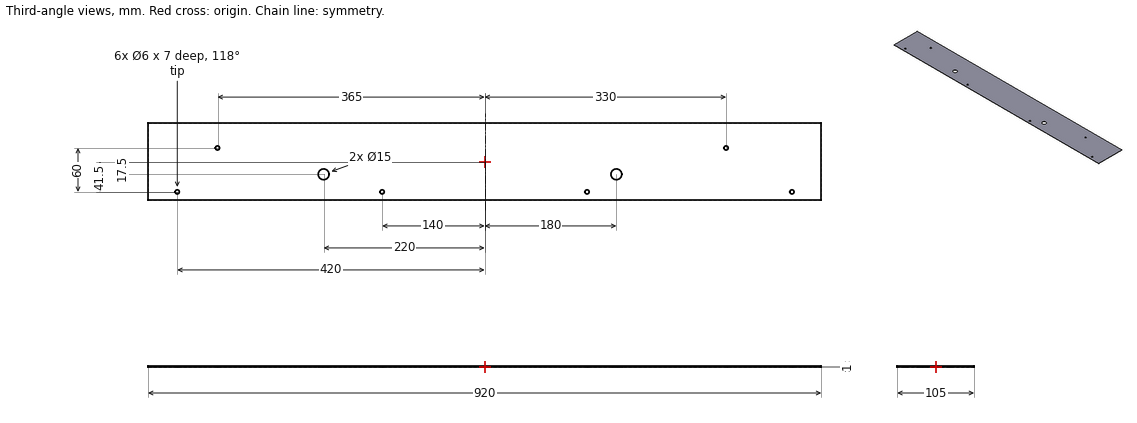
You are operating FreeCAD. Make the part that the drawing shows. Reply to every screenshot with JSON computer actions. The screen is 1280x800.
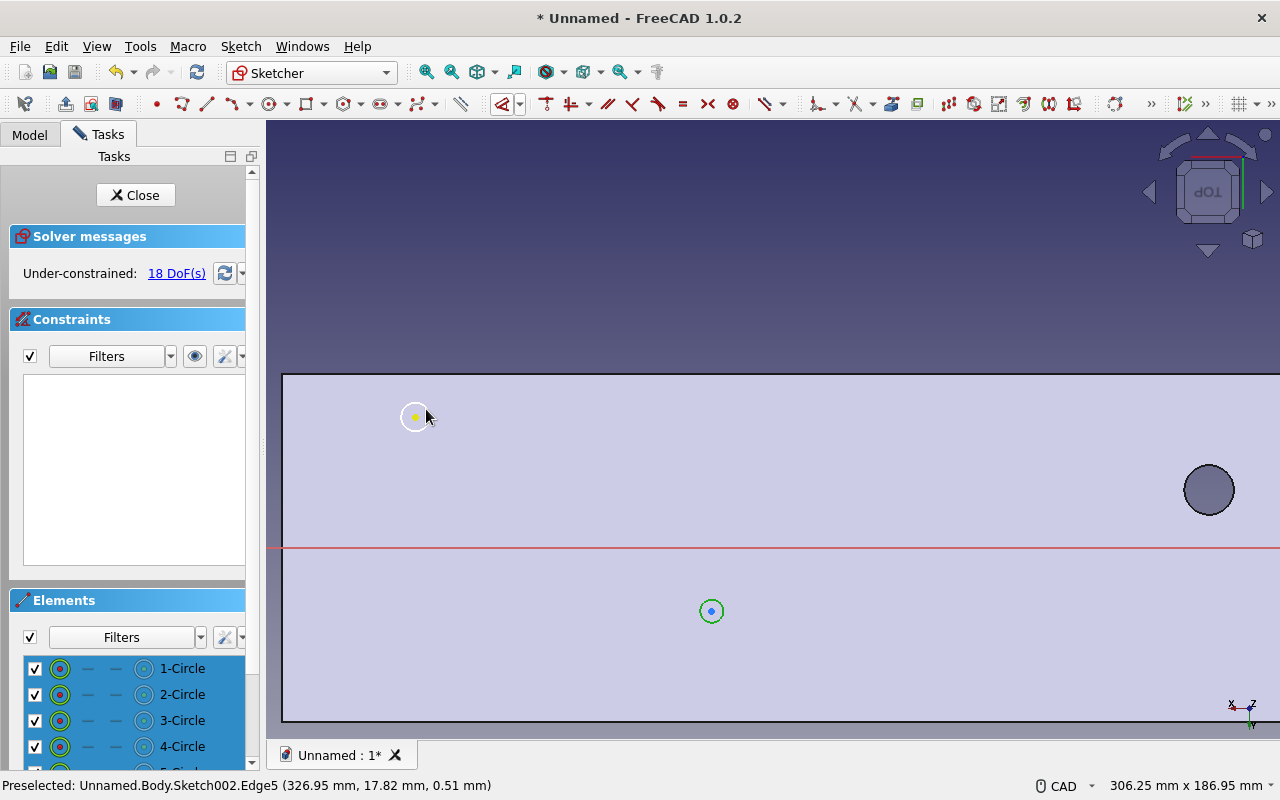
{"action": "left_click", "coordinate": [426, 407]}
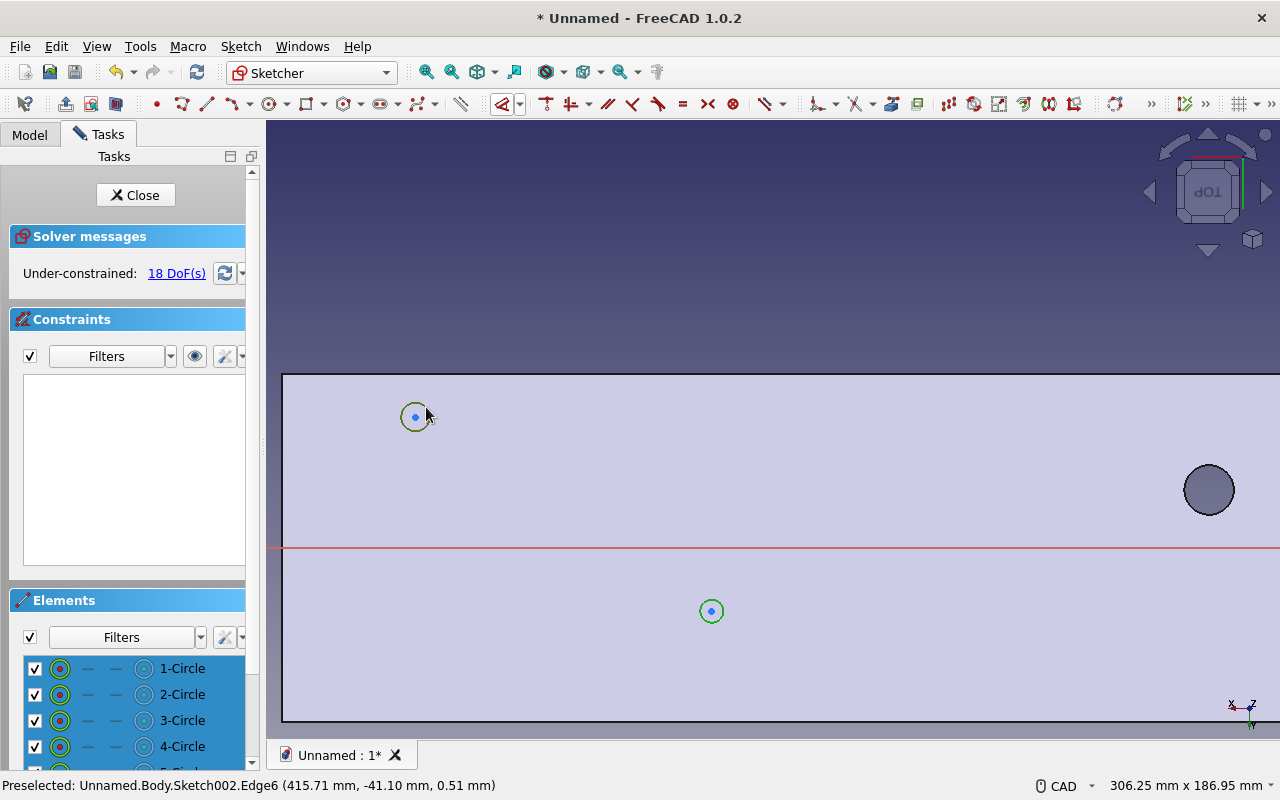
{"action": "left_click", "coordinate": [683, 104]}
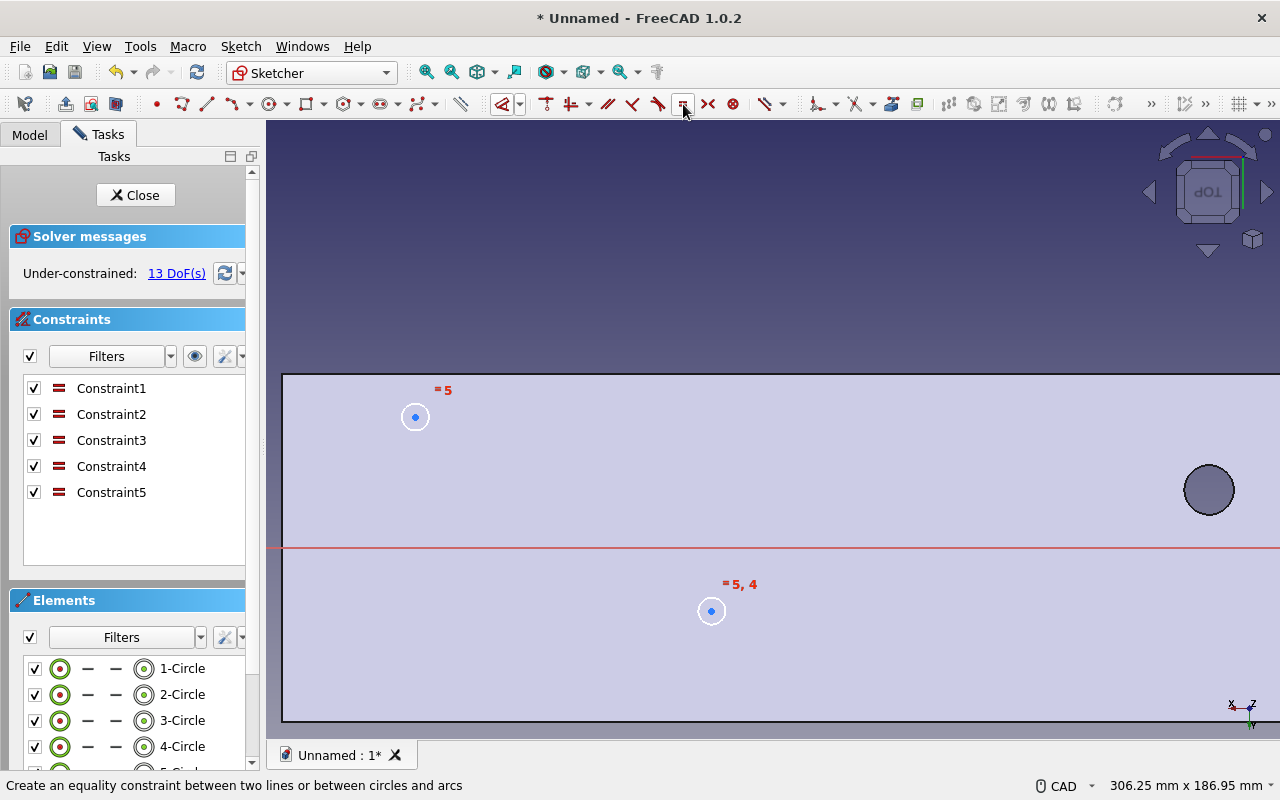
{"action": "scroll", "coordinate": [426, 409], "scroll_direction": "down", "scroll_amount": 8}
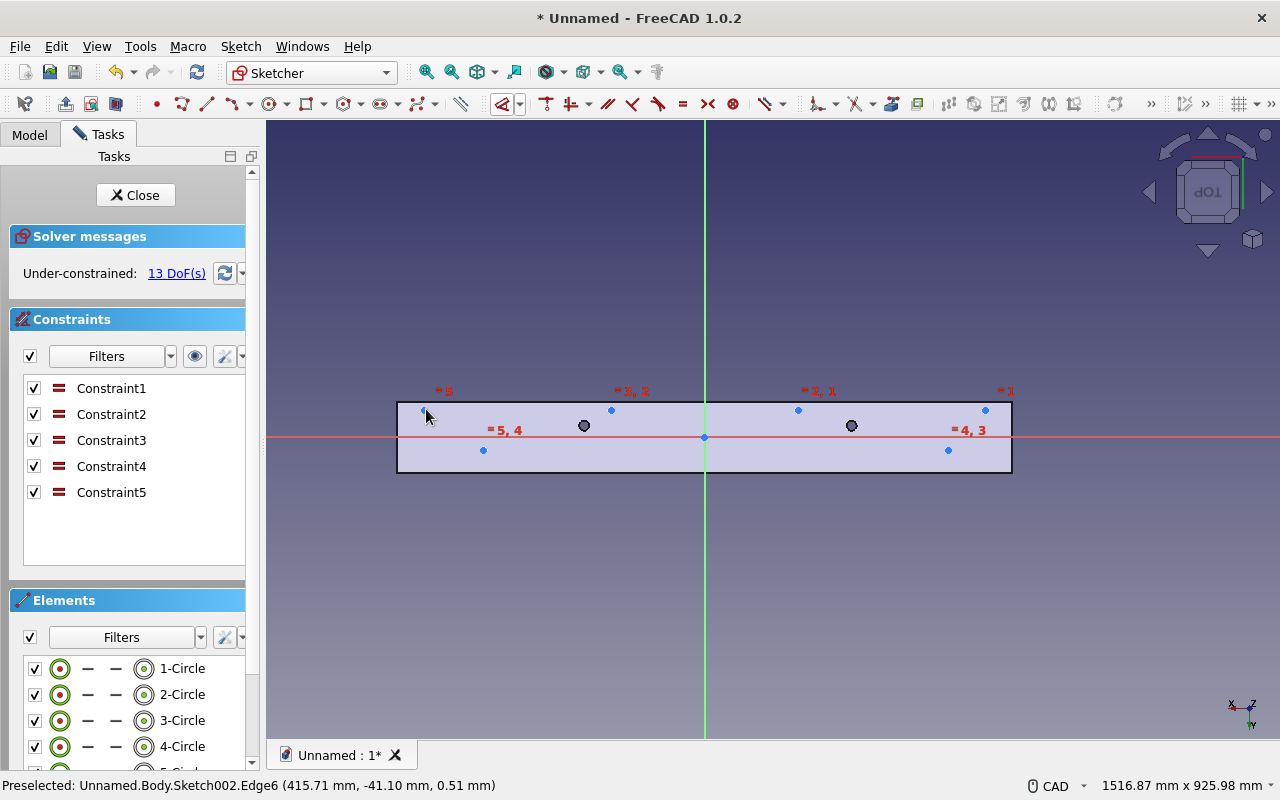
{"action": "left_click", "coordinate": [798, 411]}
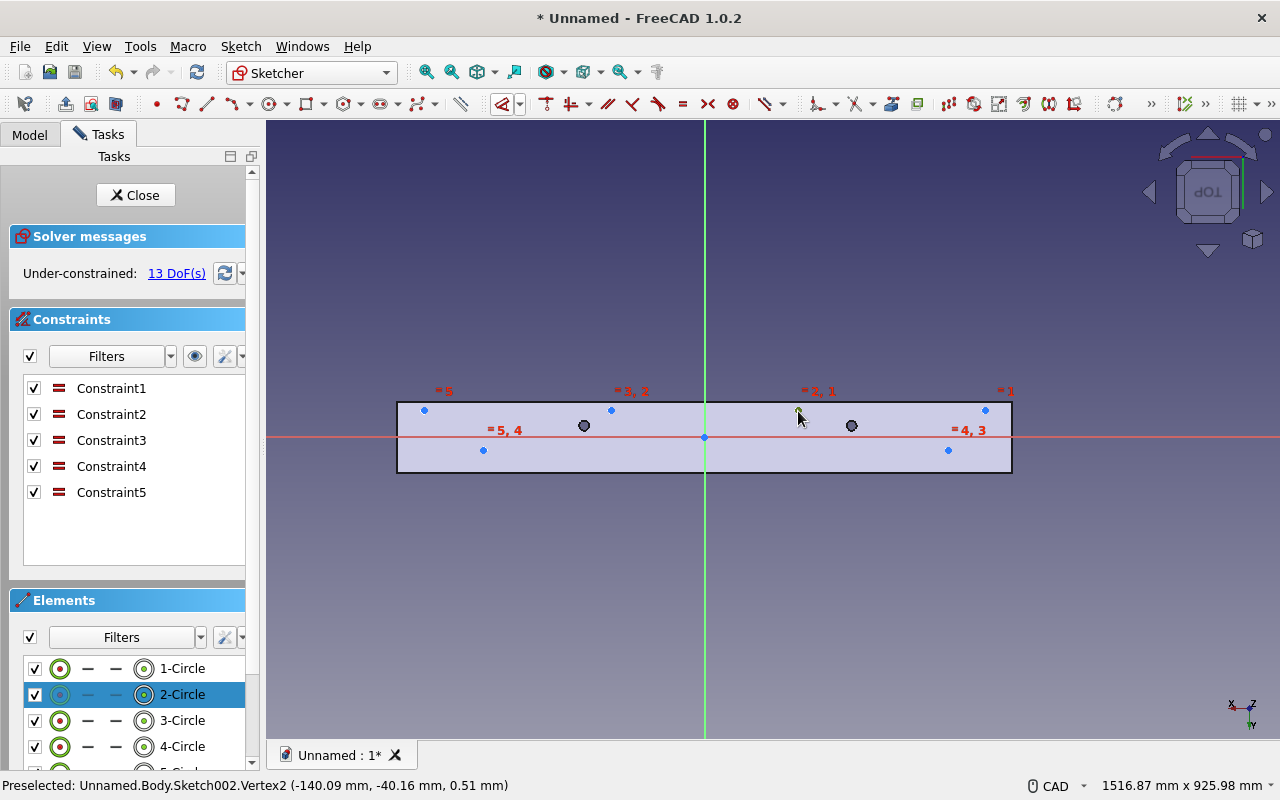
{"action": "left_click", "coordinate": [611, 411]}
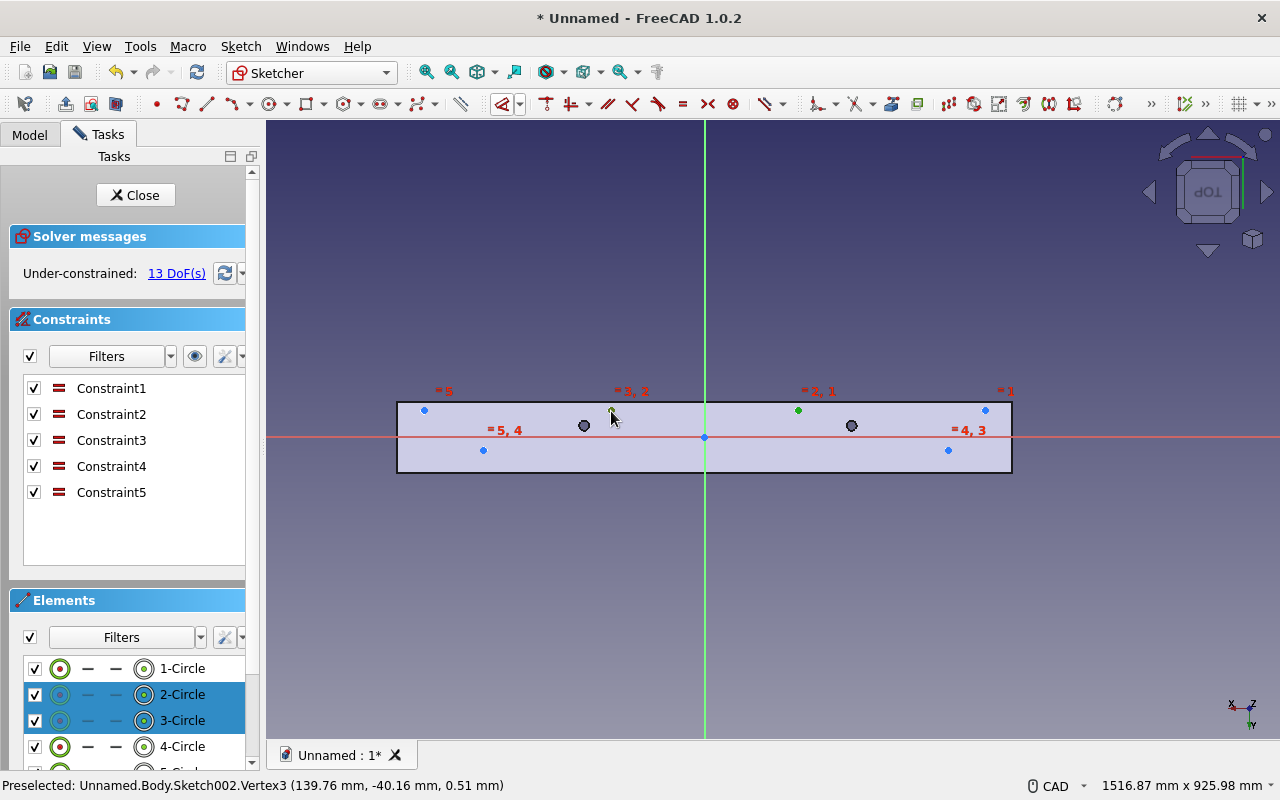
{"action": "left_click", "coordinate": [705, 671]}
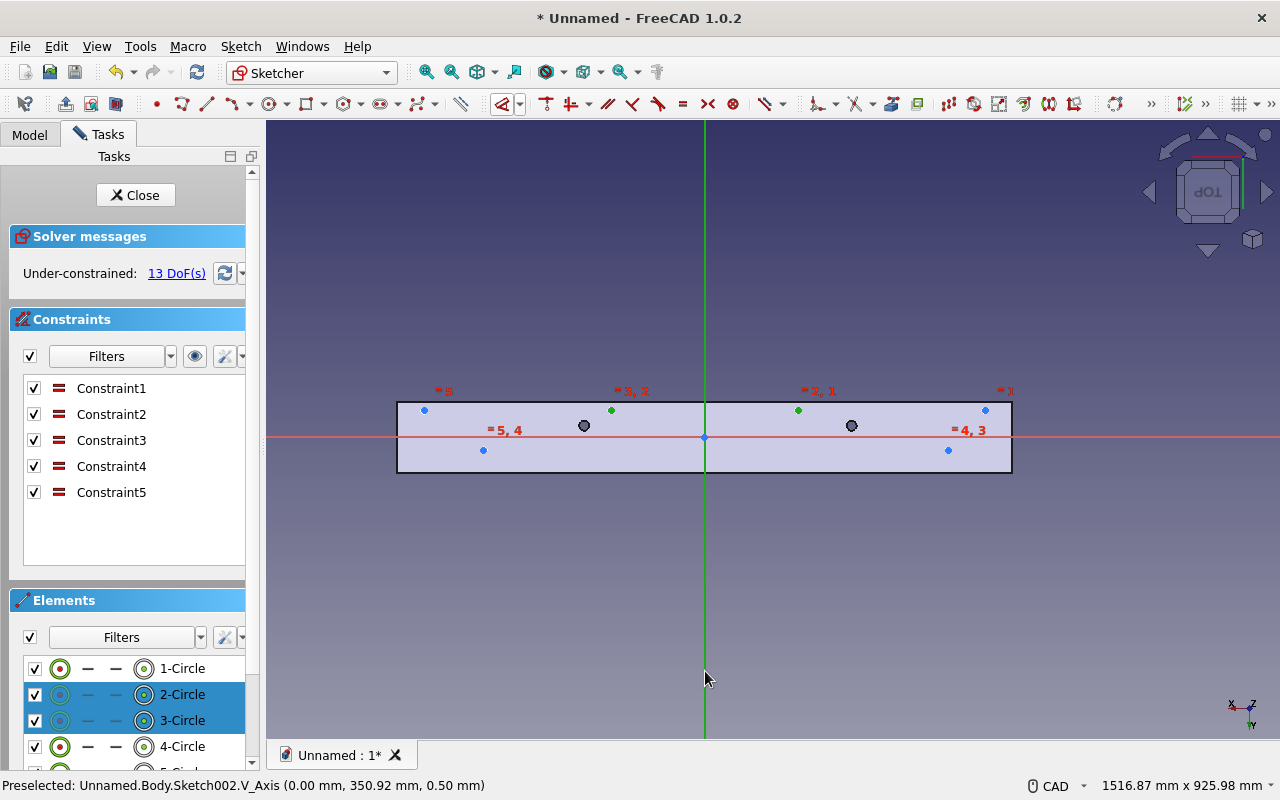
{"action": "left_click", "coordinate": [708, 104]}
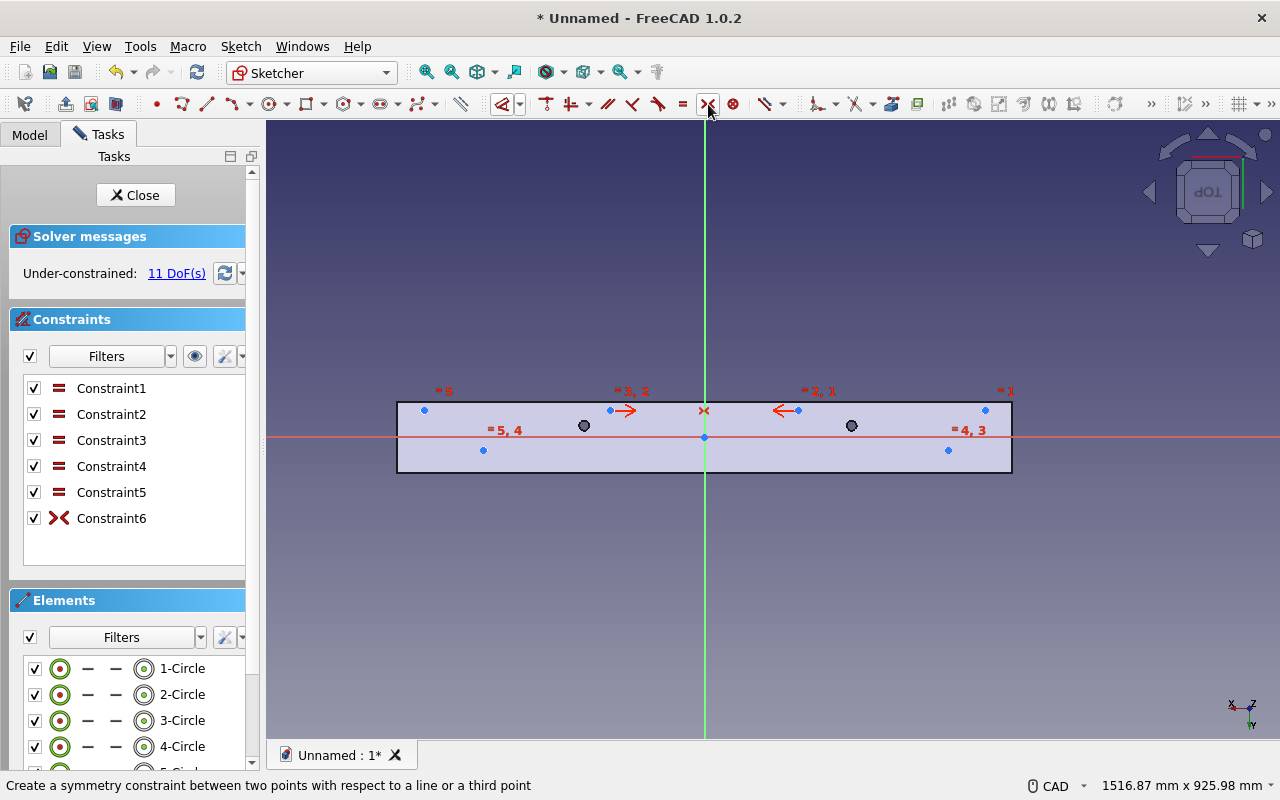
{"action": "left_click", "coordinate": [985, 411]}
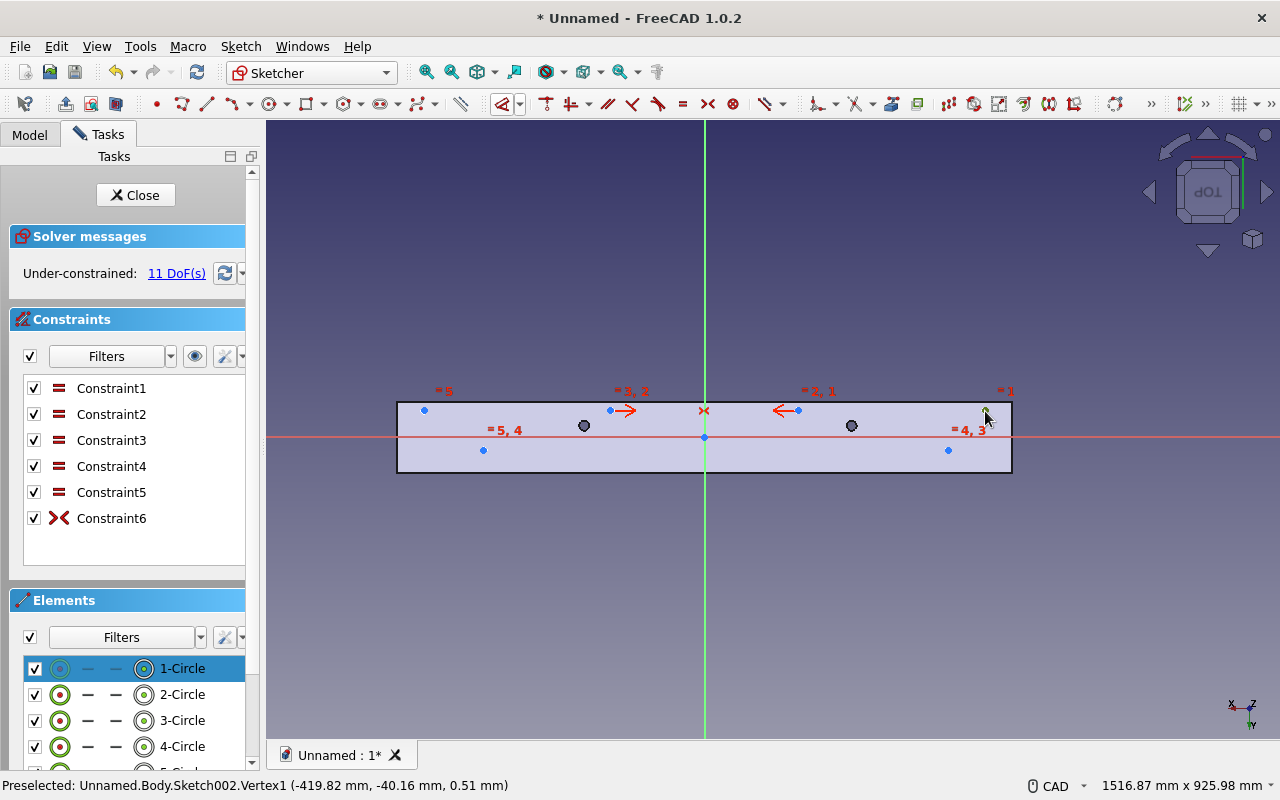
{"action": "left_click", "coordinate": [424, 411]}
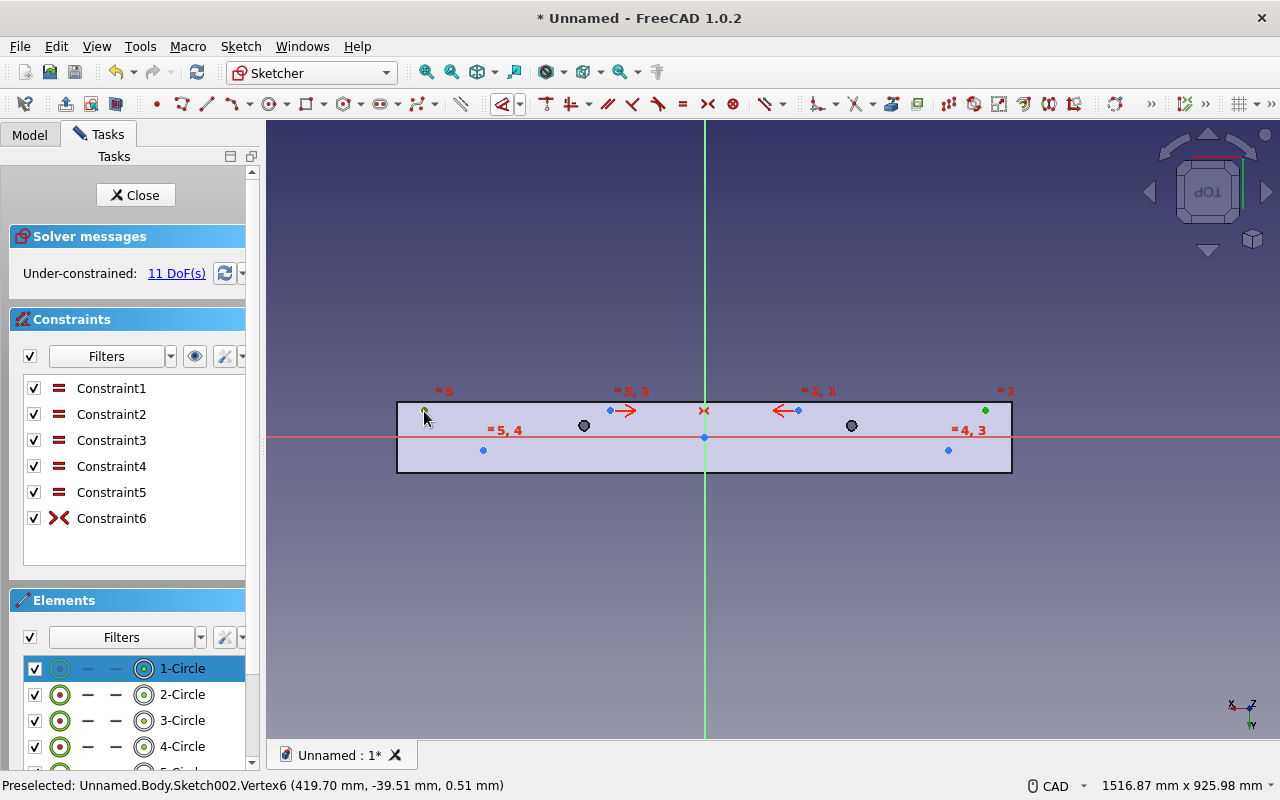
{"action": "left_click", "coordinate": [705, 671]}